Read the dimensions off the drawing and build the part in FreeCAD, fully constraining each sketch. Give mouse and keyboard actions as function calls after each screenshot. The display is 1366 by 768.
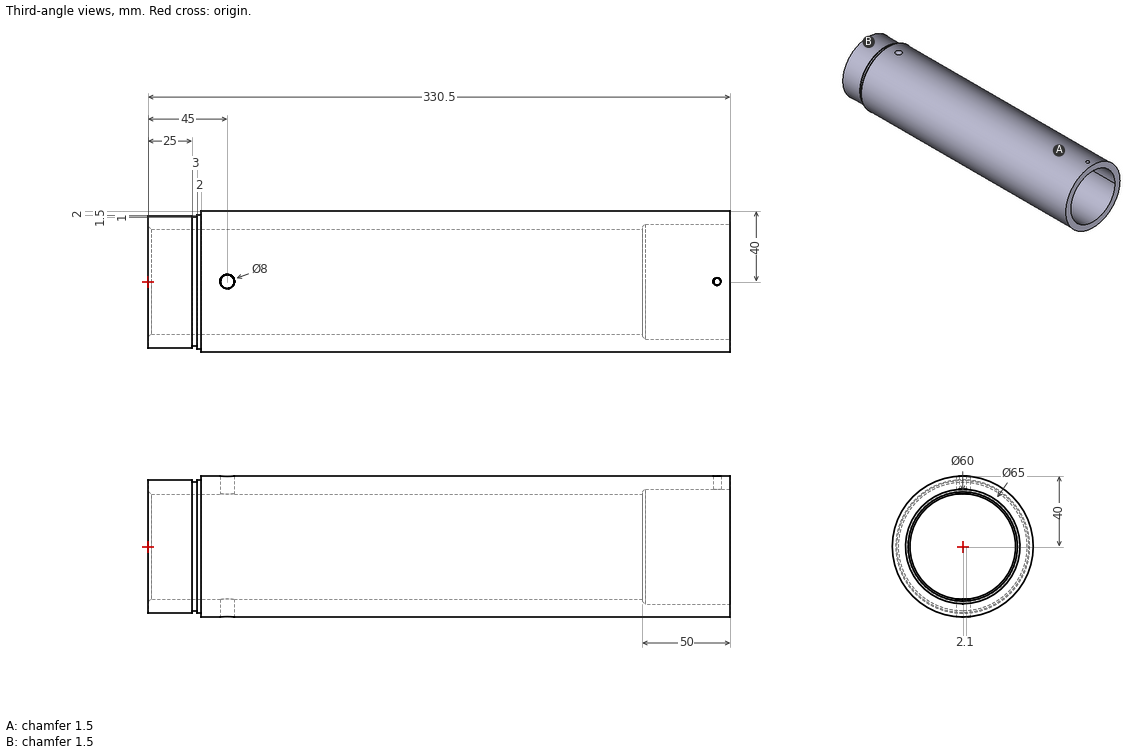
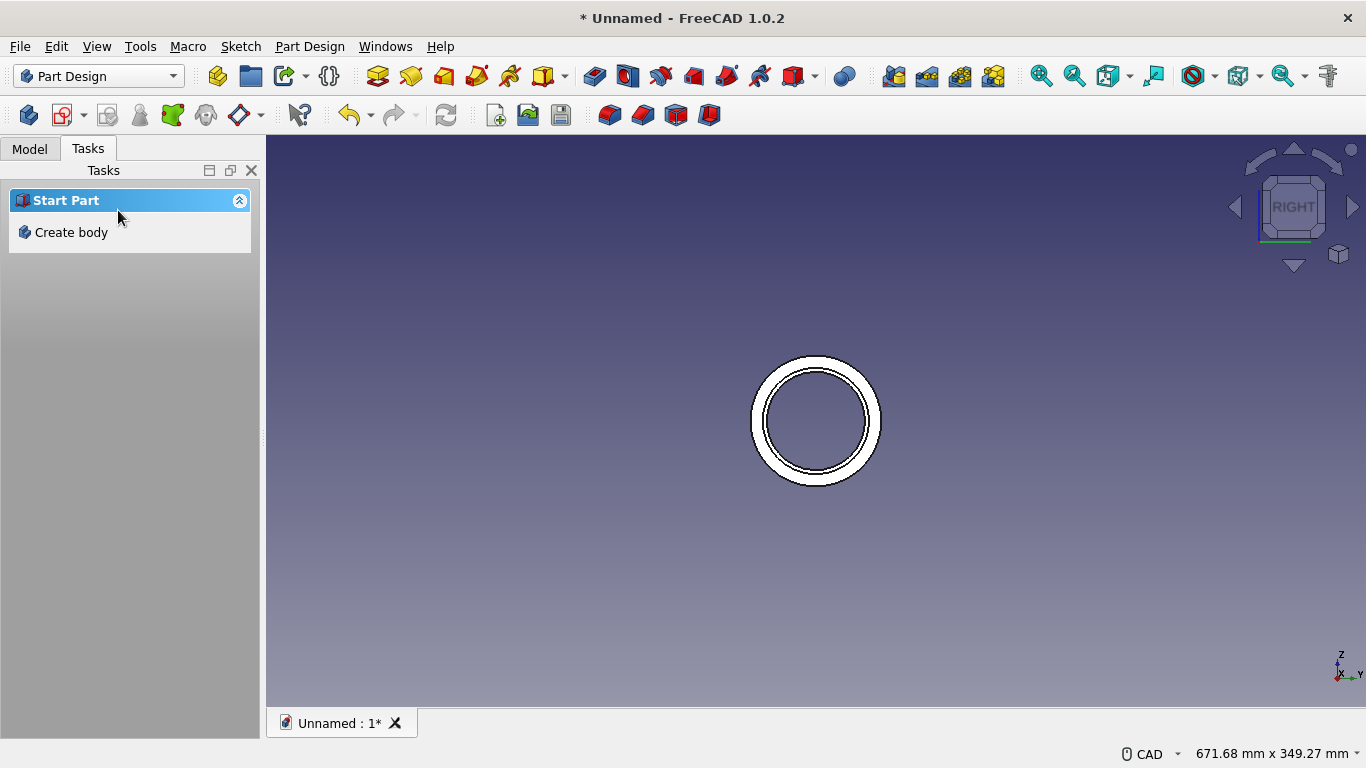
click(1042, 76)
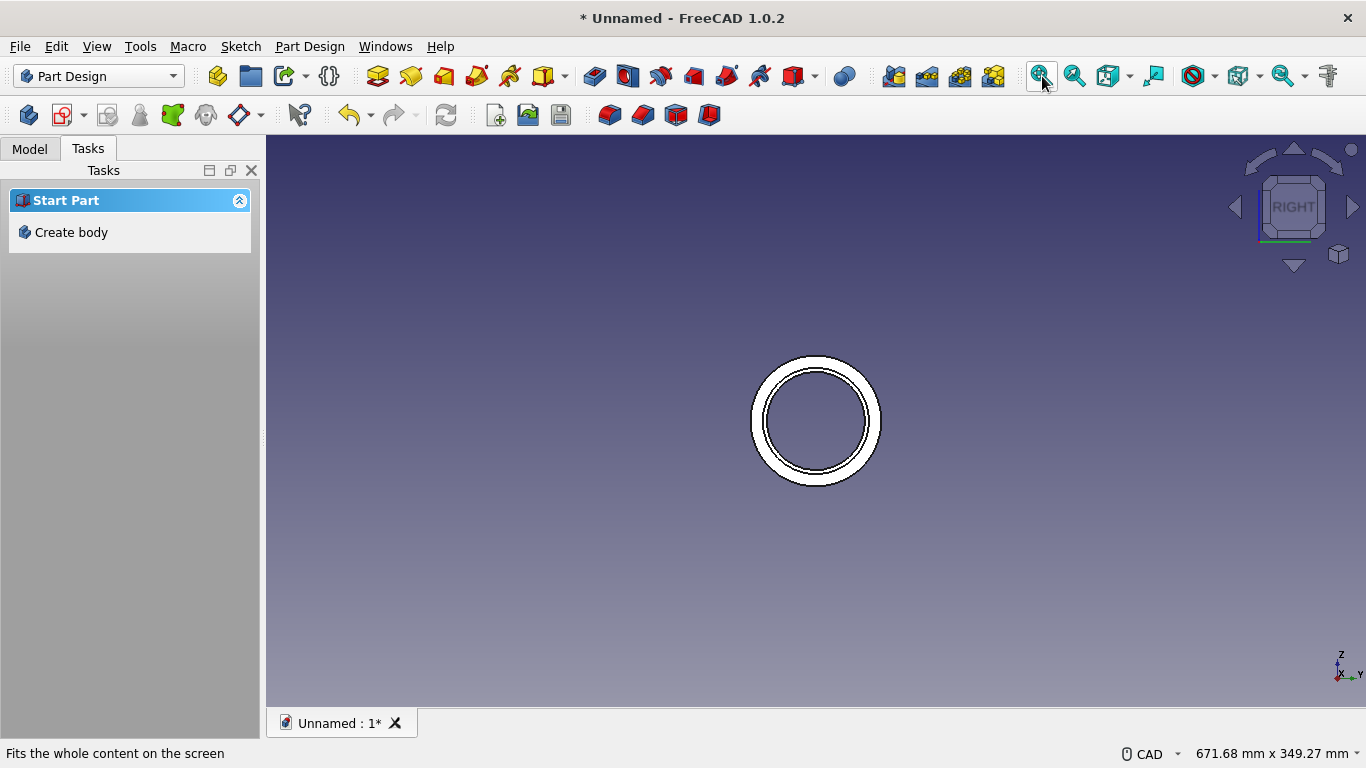
key(0)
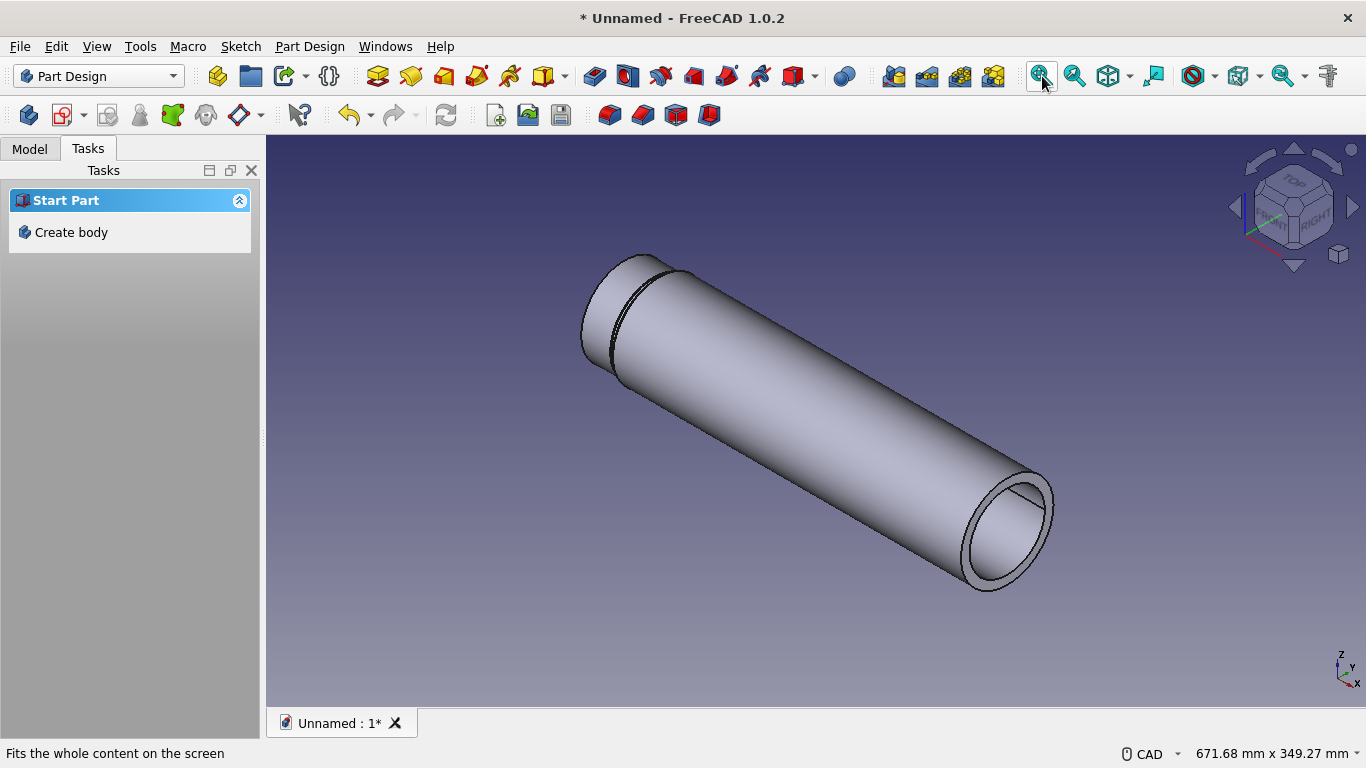
key(2)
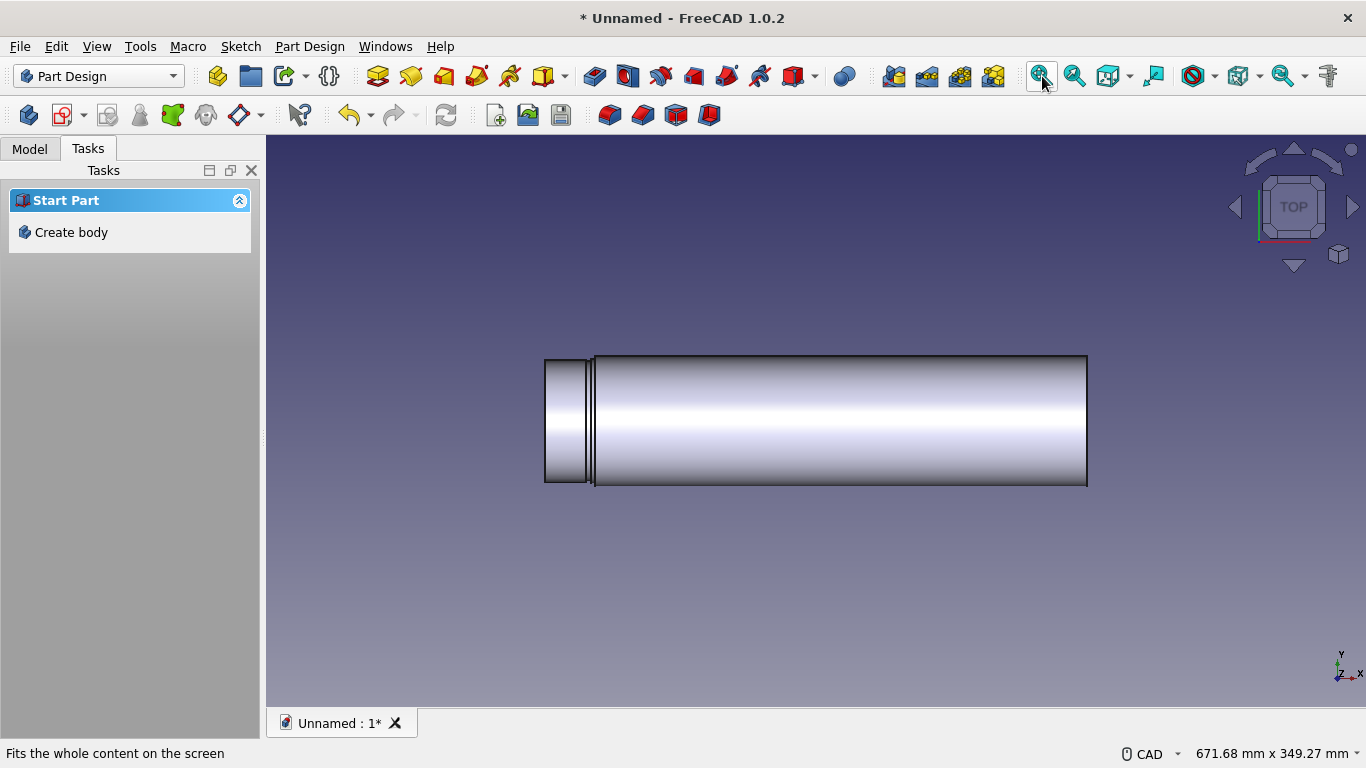
key(1)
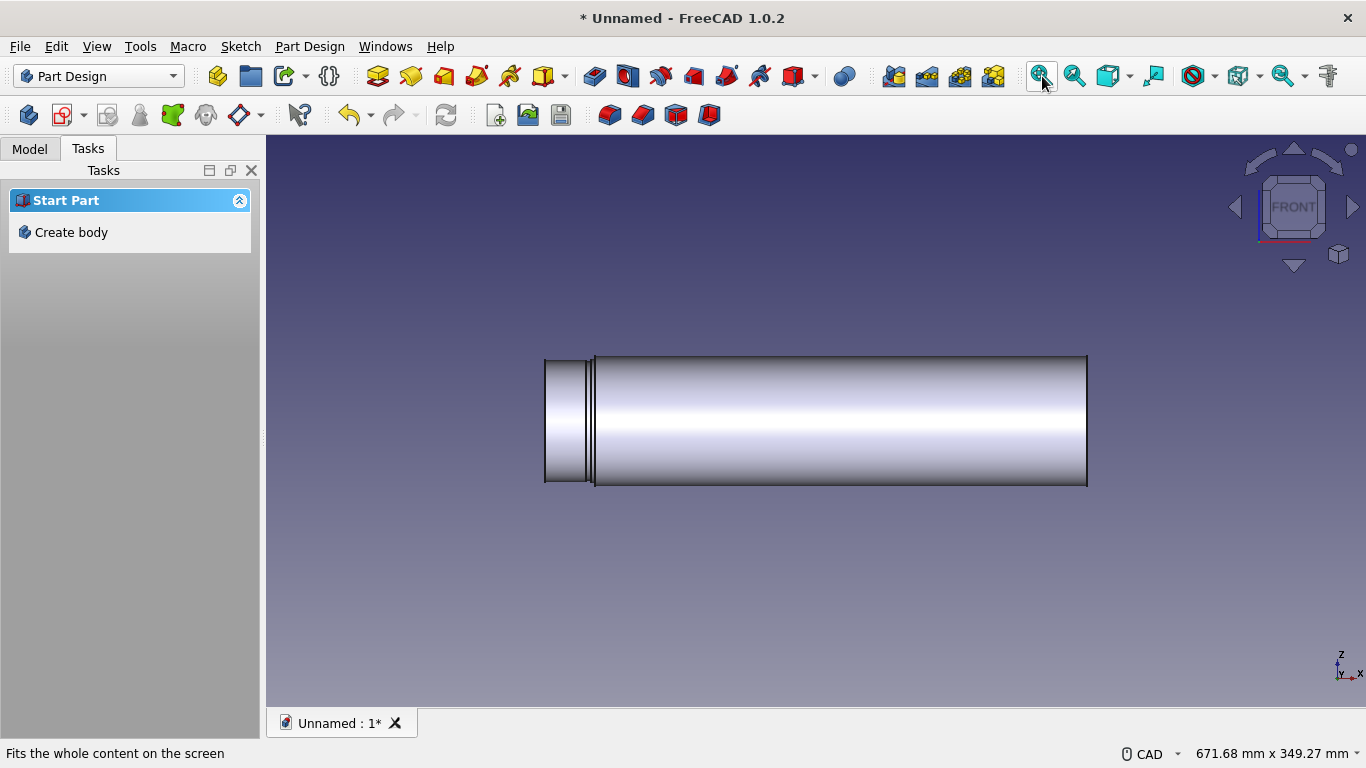
key(3)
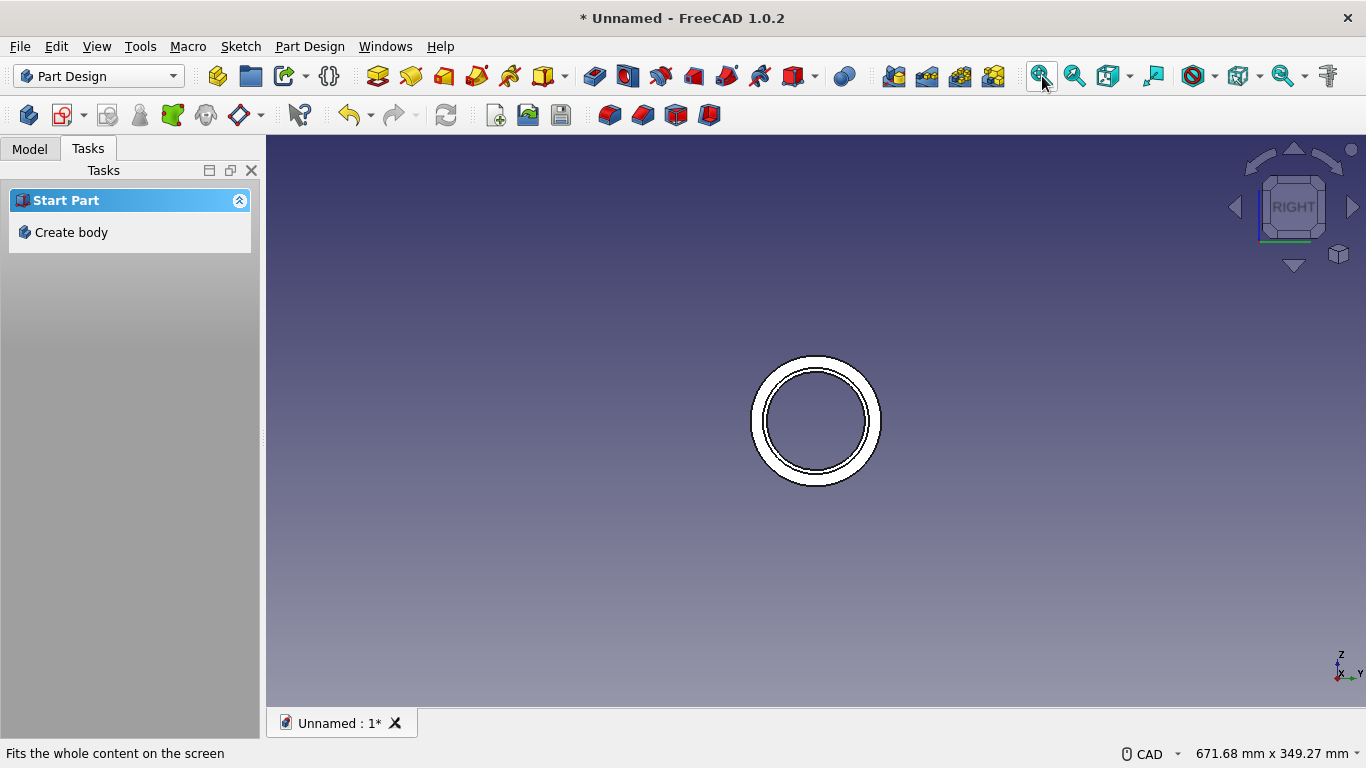
click(1042, 76)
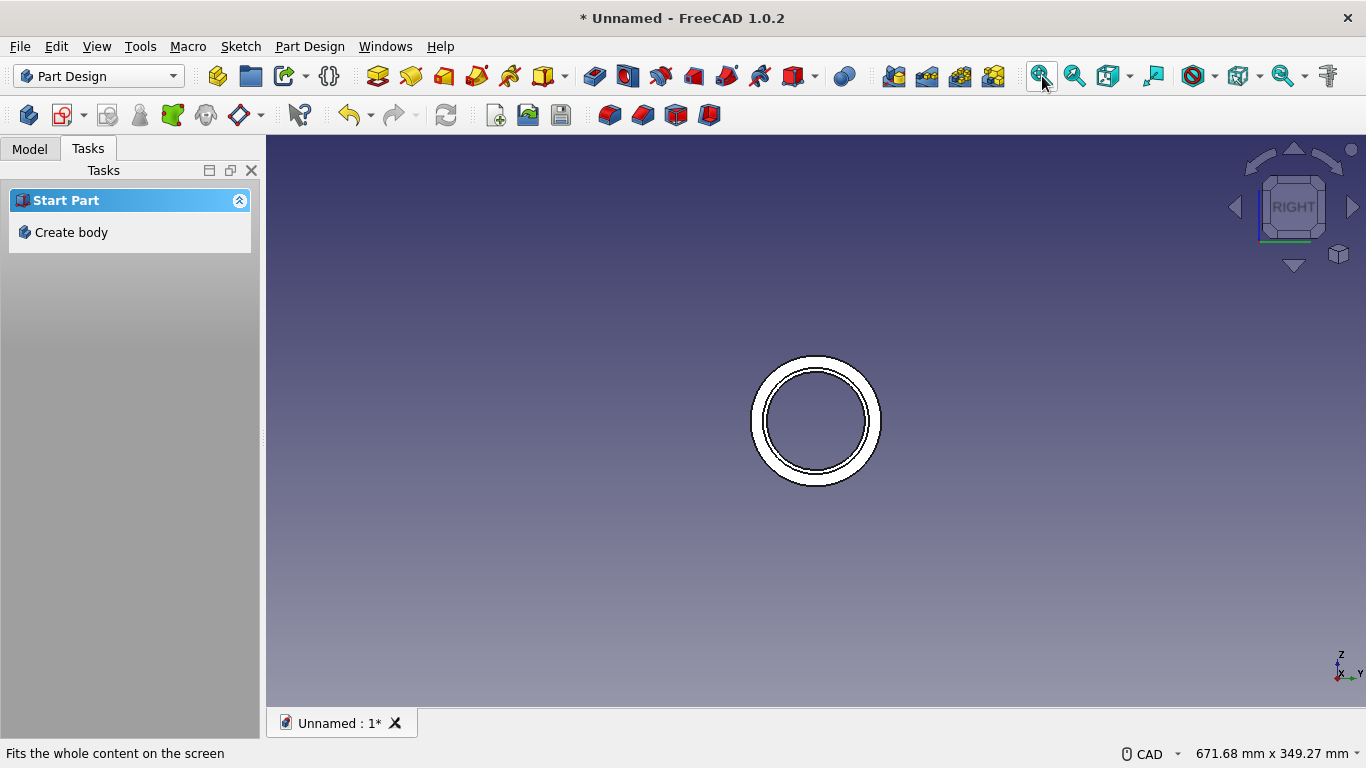
key(5)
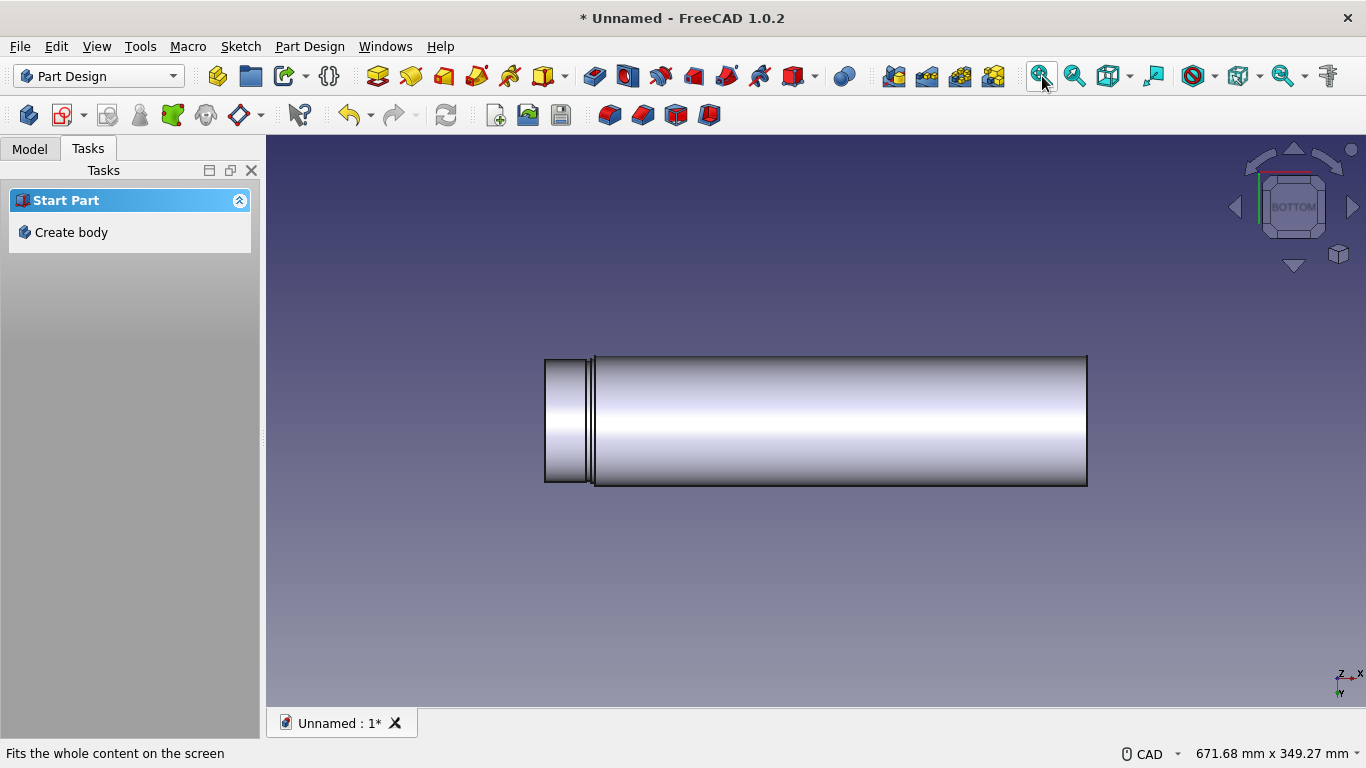
key(4)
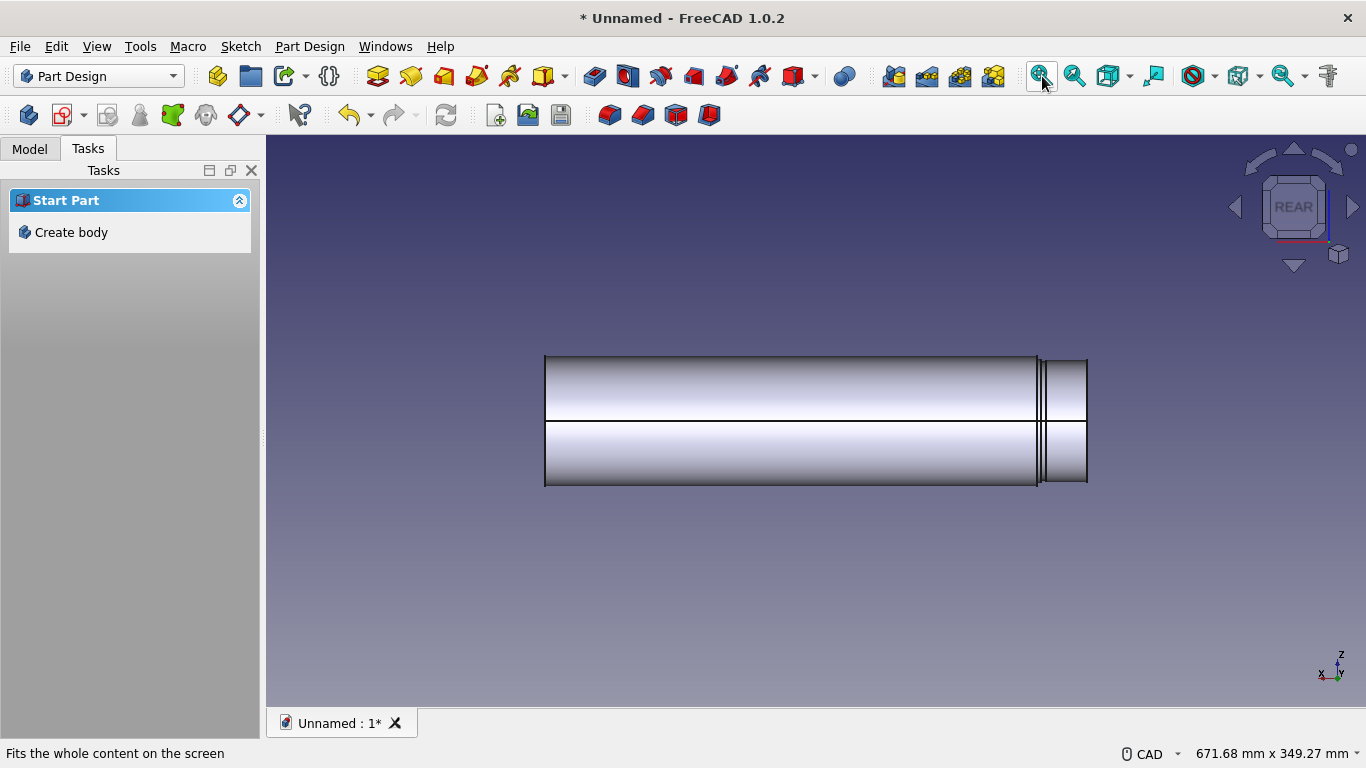
key(6)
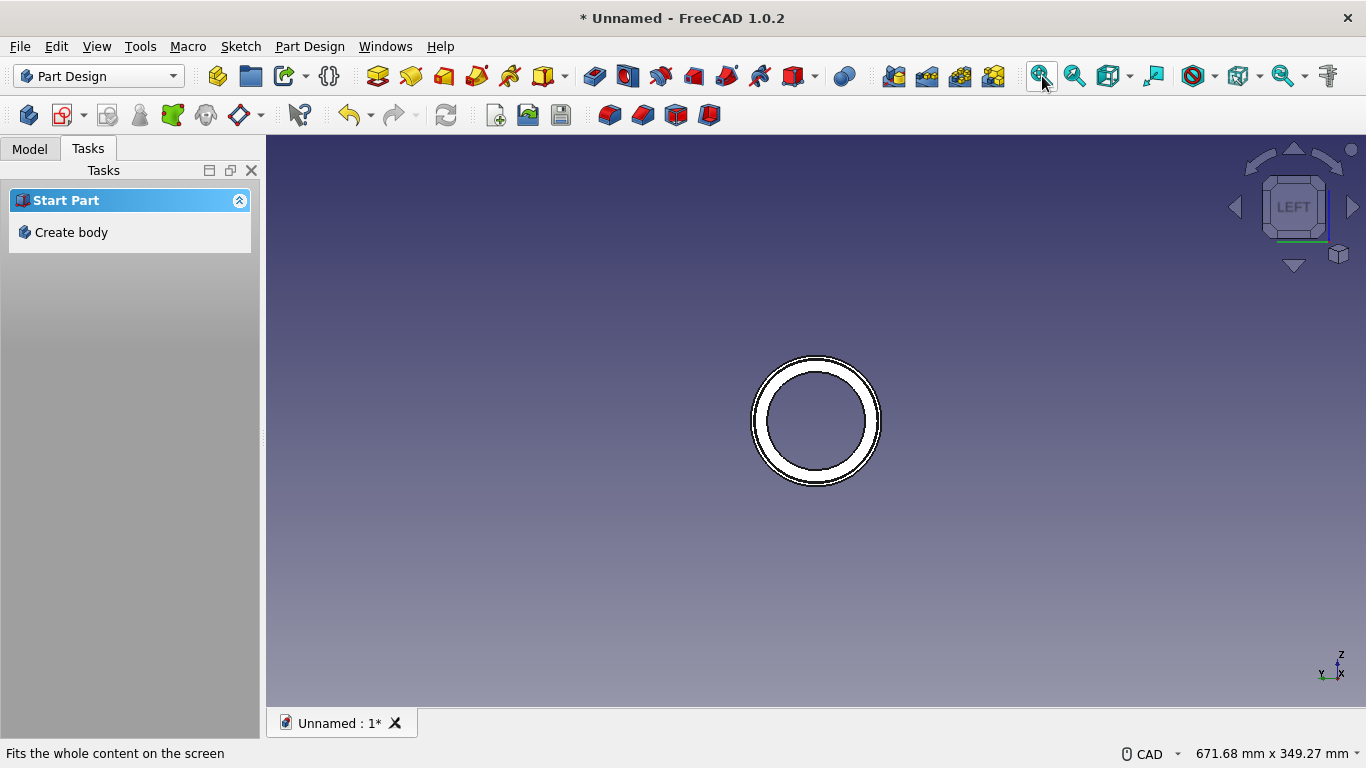
click(1042, 76)